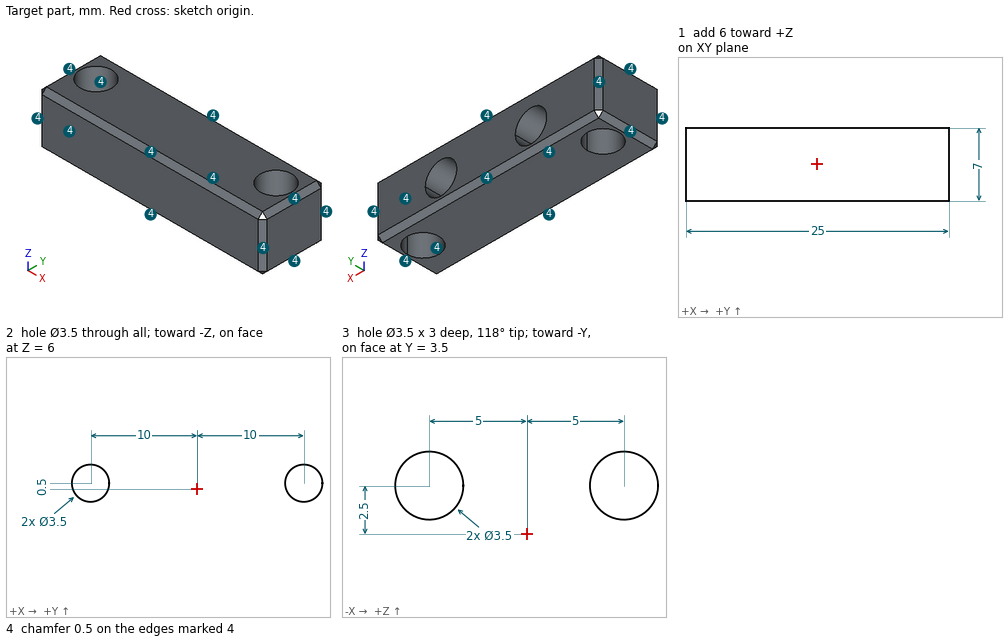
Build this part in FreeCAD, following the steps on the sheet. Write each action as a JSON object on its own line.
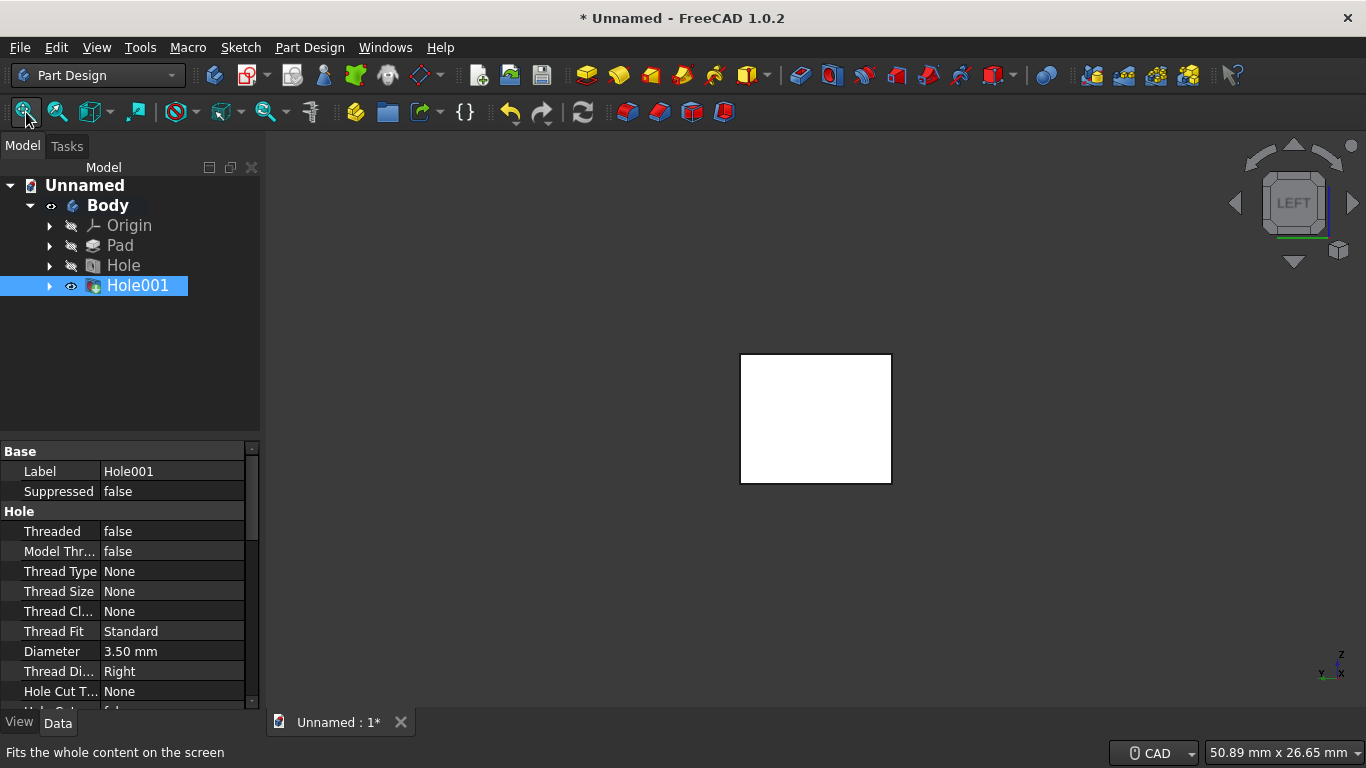
{"action": "left_click", "coordinate": [816, 418], "text": "ctrl"}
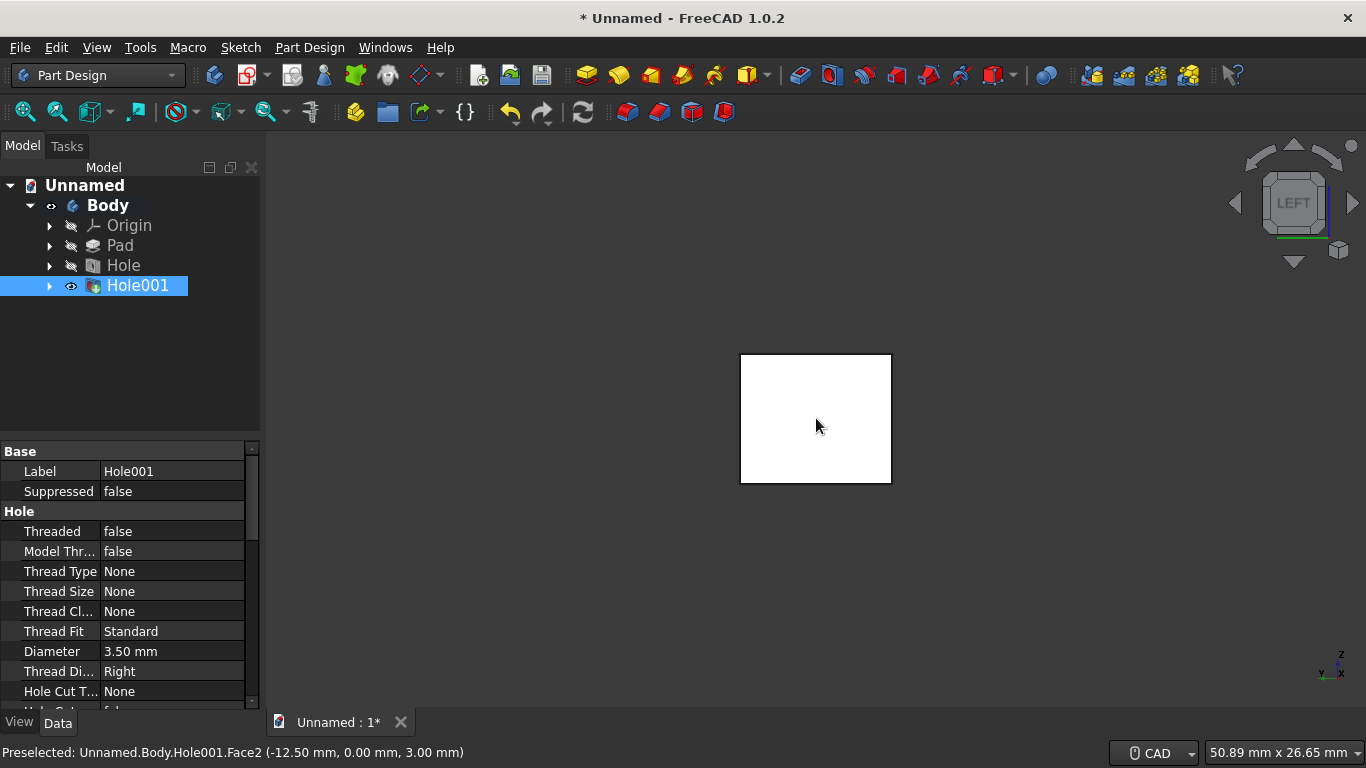
{"action": "left_click", "coordinate": [660, 112]}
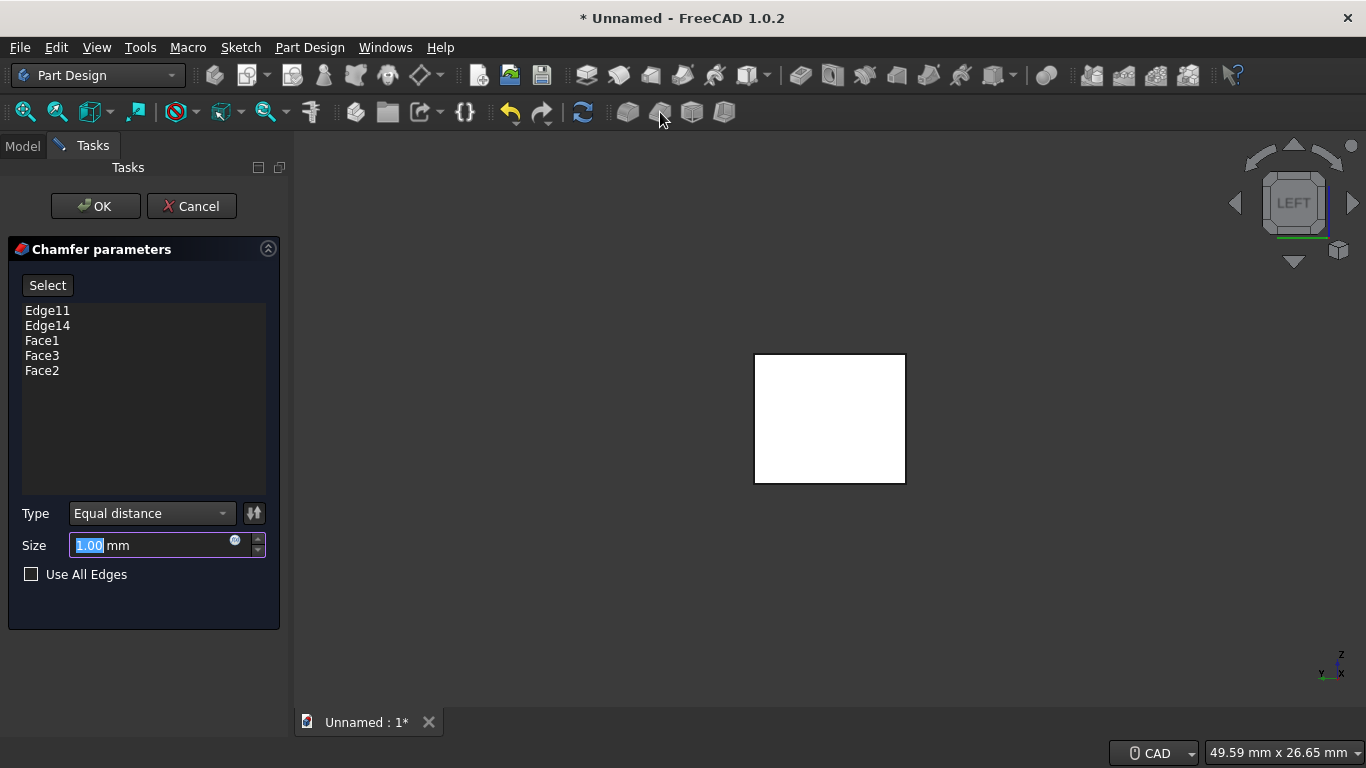
{"action": "type", "text": "0.5"}
{"action": "key", "text": "Tab"}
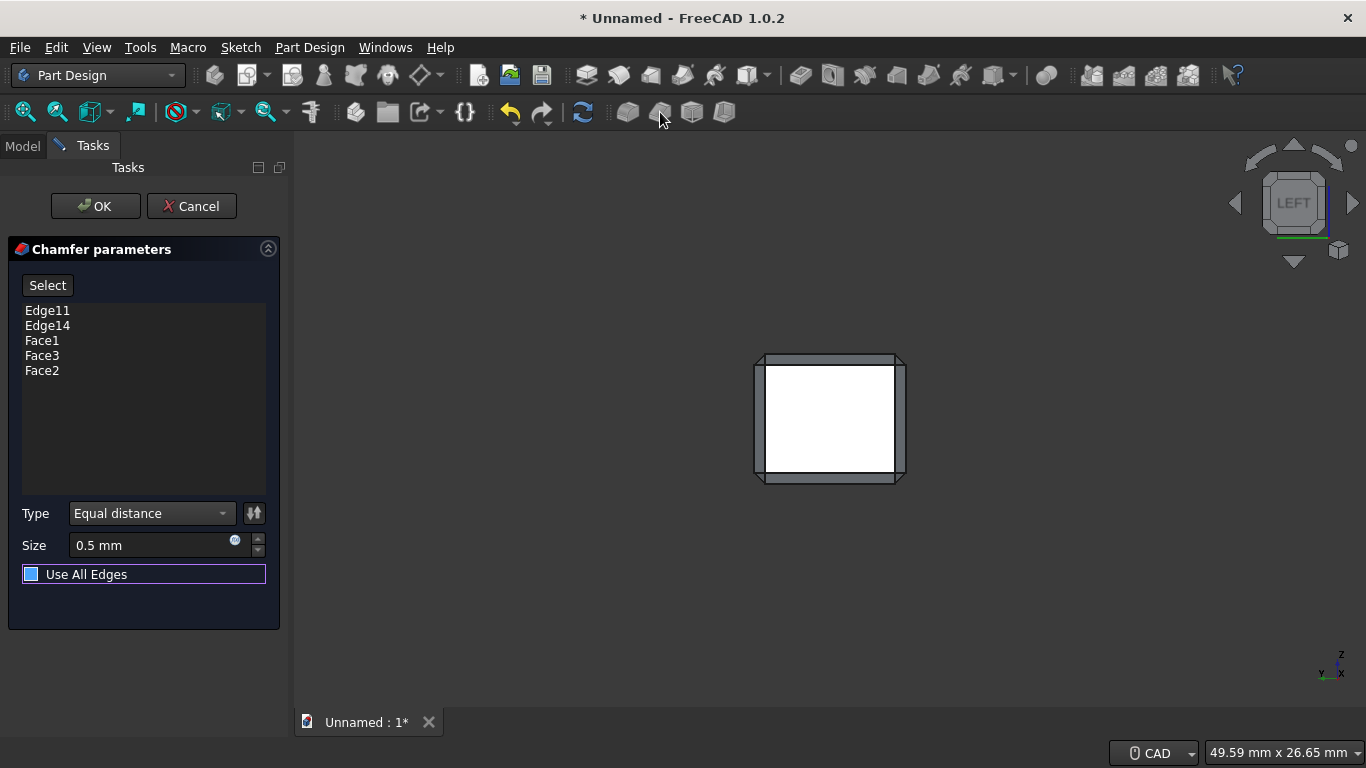
{"action": "left_click", "coordinate": [96, 206]}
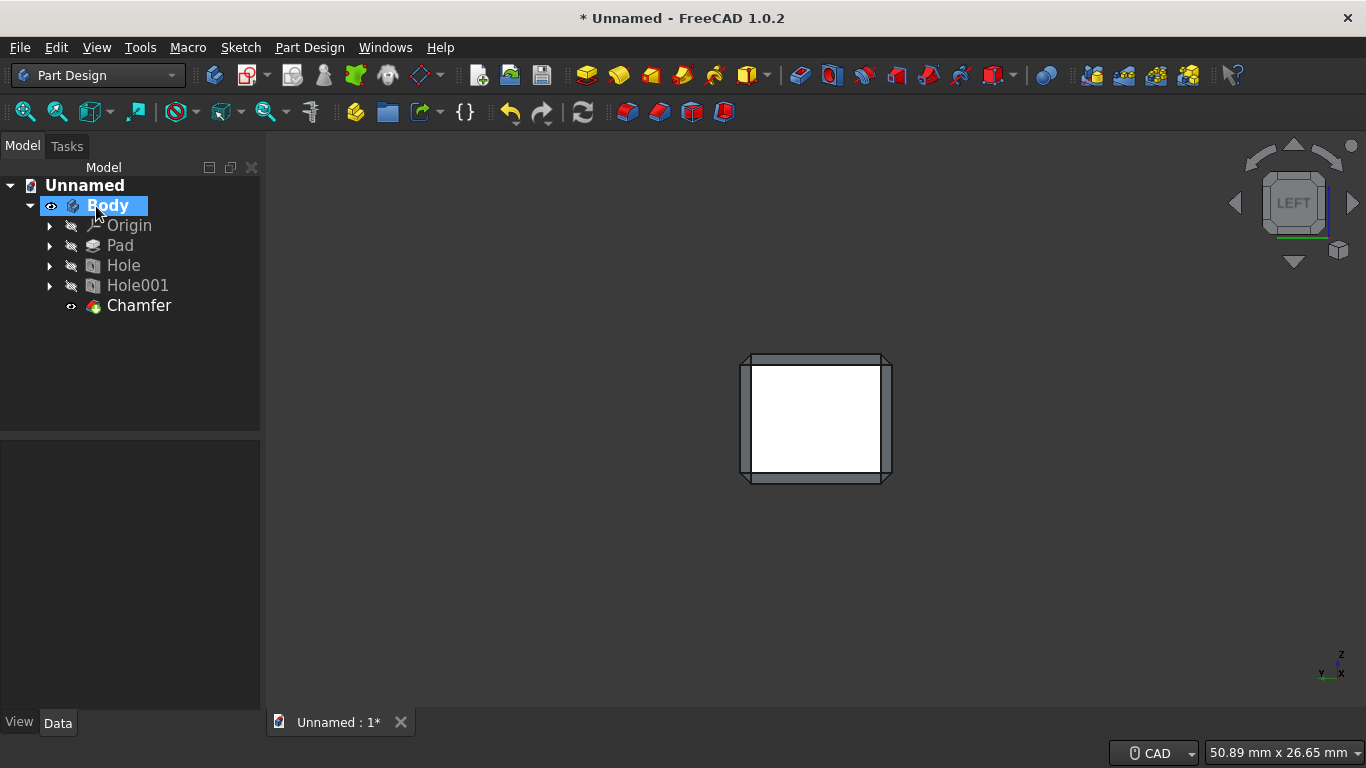
{"action": "key", "text": "0"}